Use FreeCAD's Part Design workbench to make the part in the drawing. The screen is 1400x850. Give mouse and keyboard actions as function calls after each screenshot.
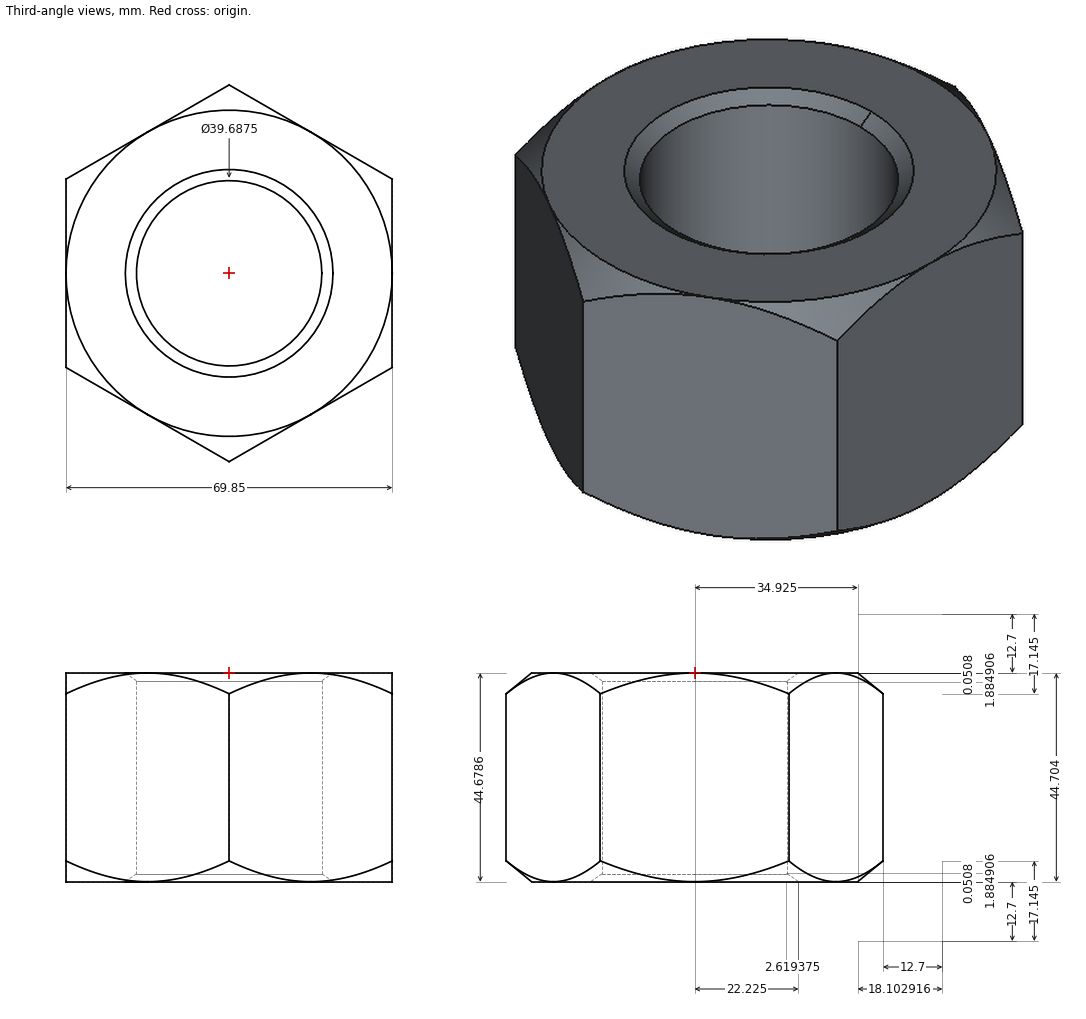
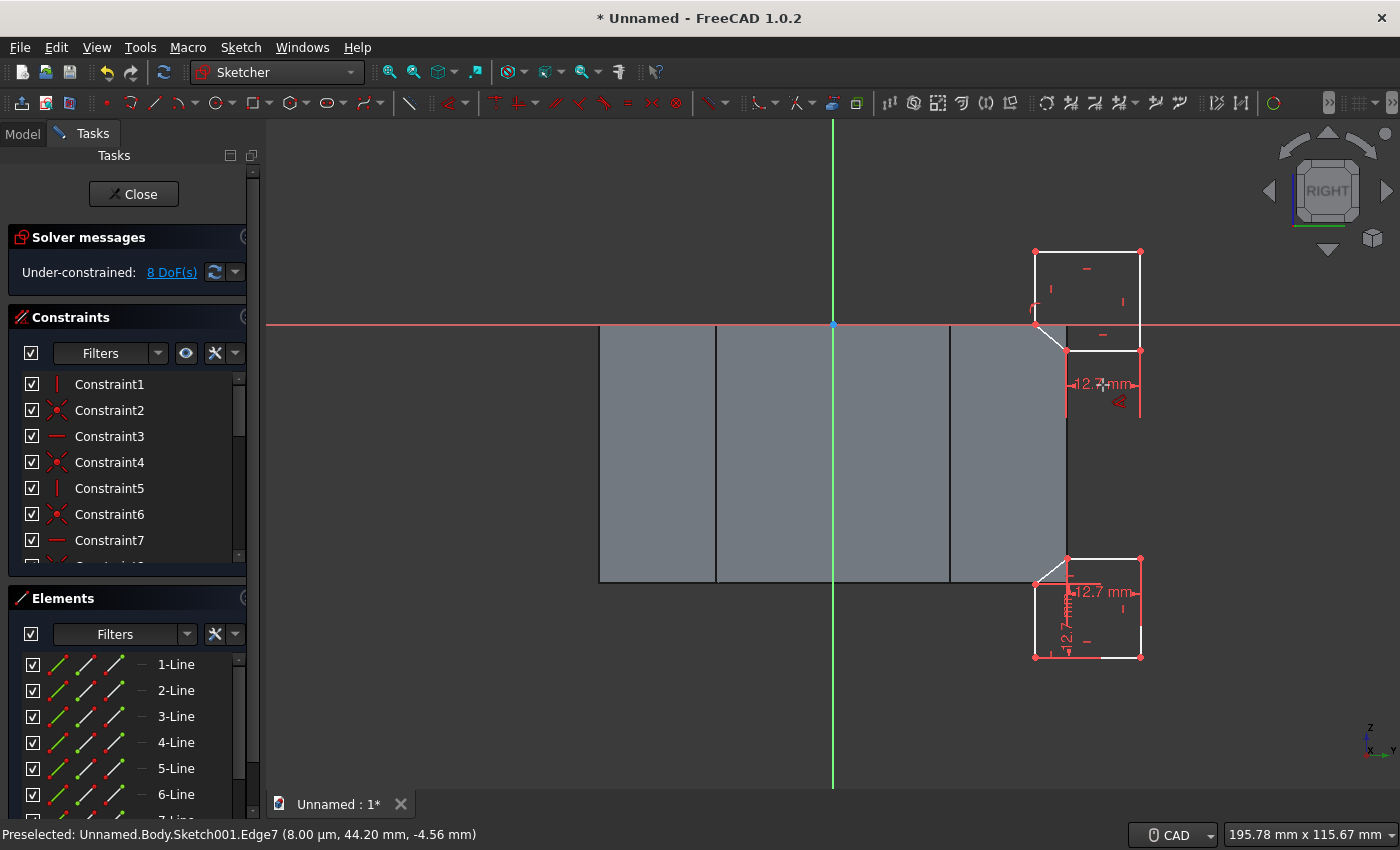
click(1035, 274)
click(1069, 288)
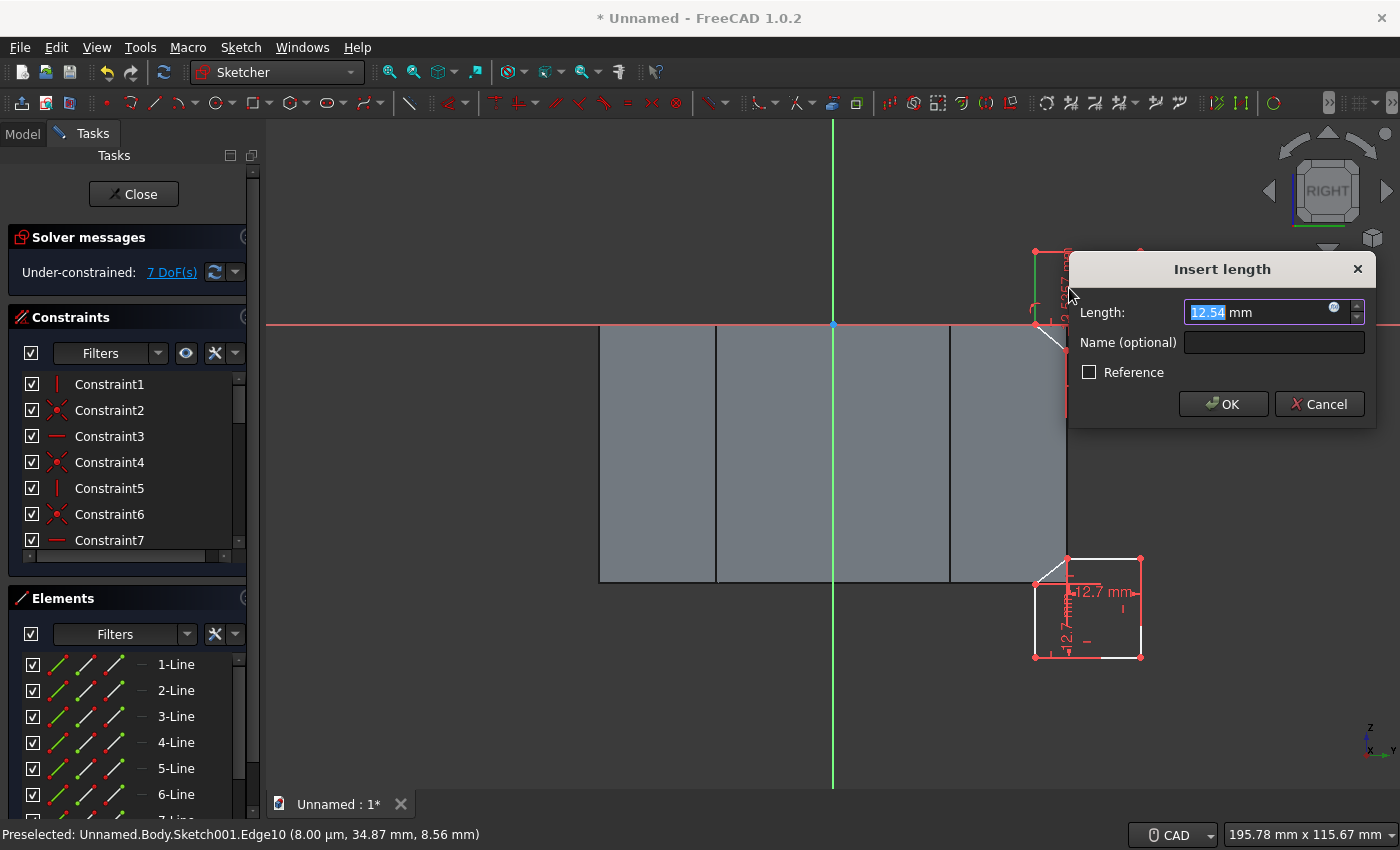
text(12.7)
key(Return)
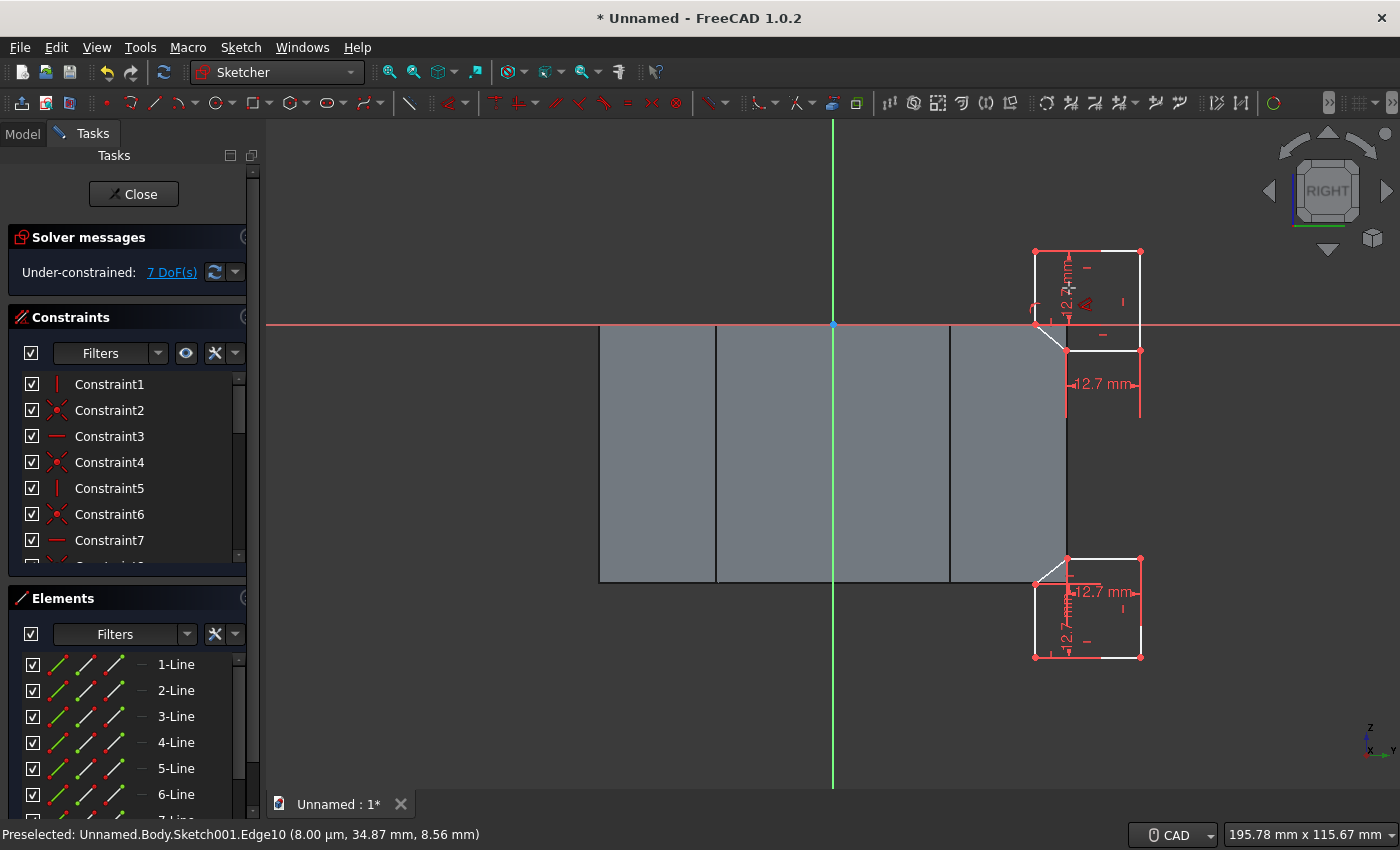
click(1141, 628)
click(1175, 608)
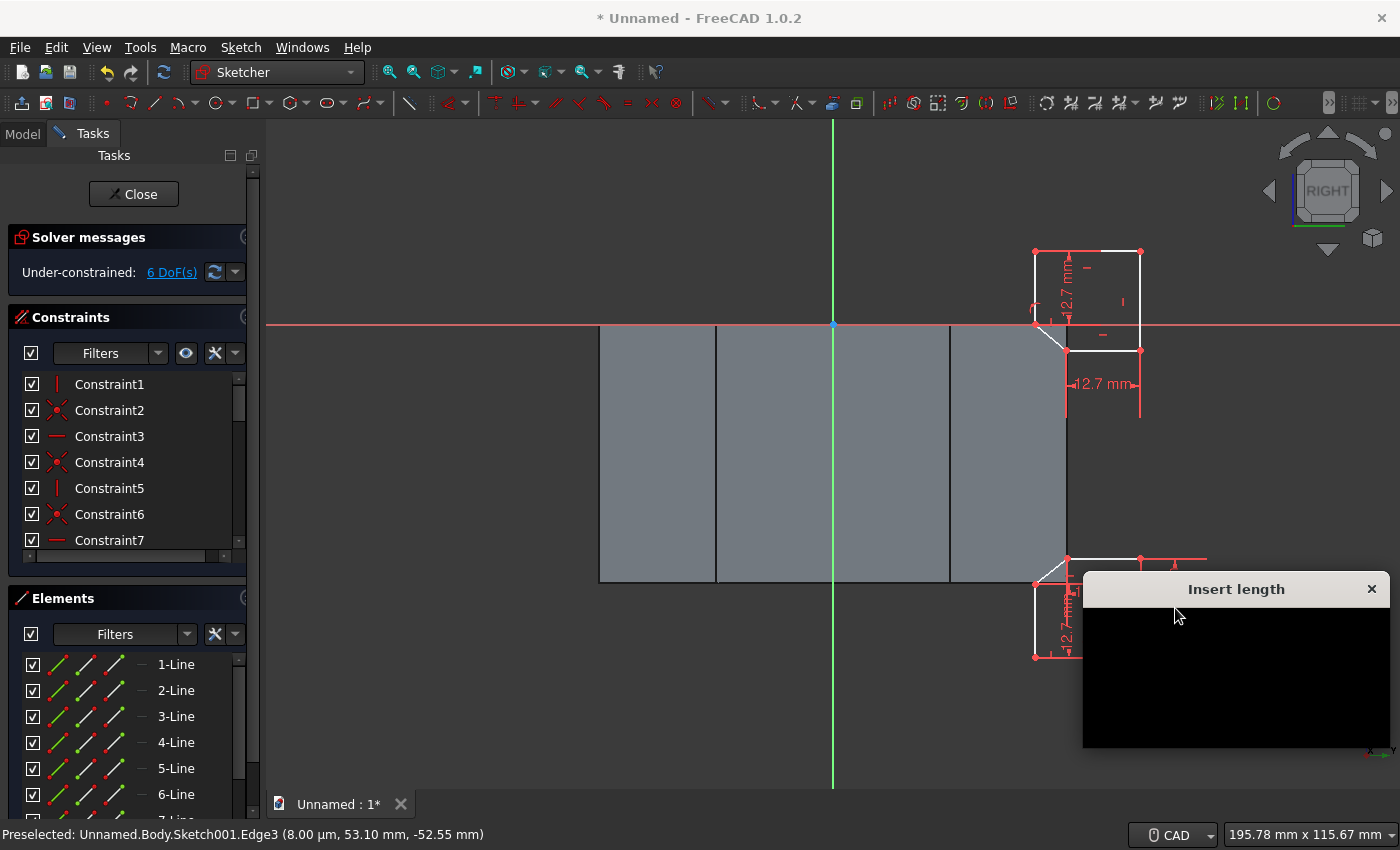
text(17.145)
key(Return)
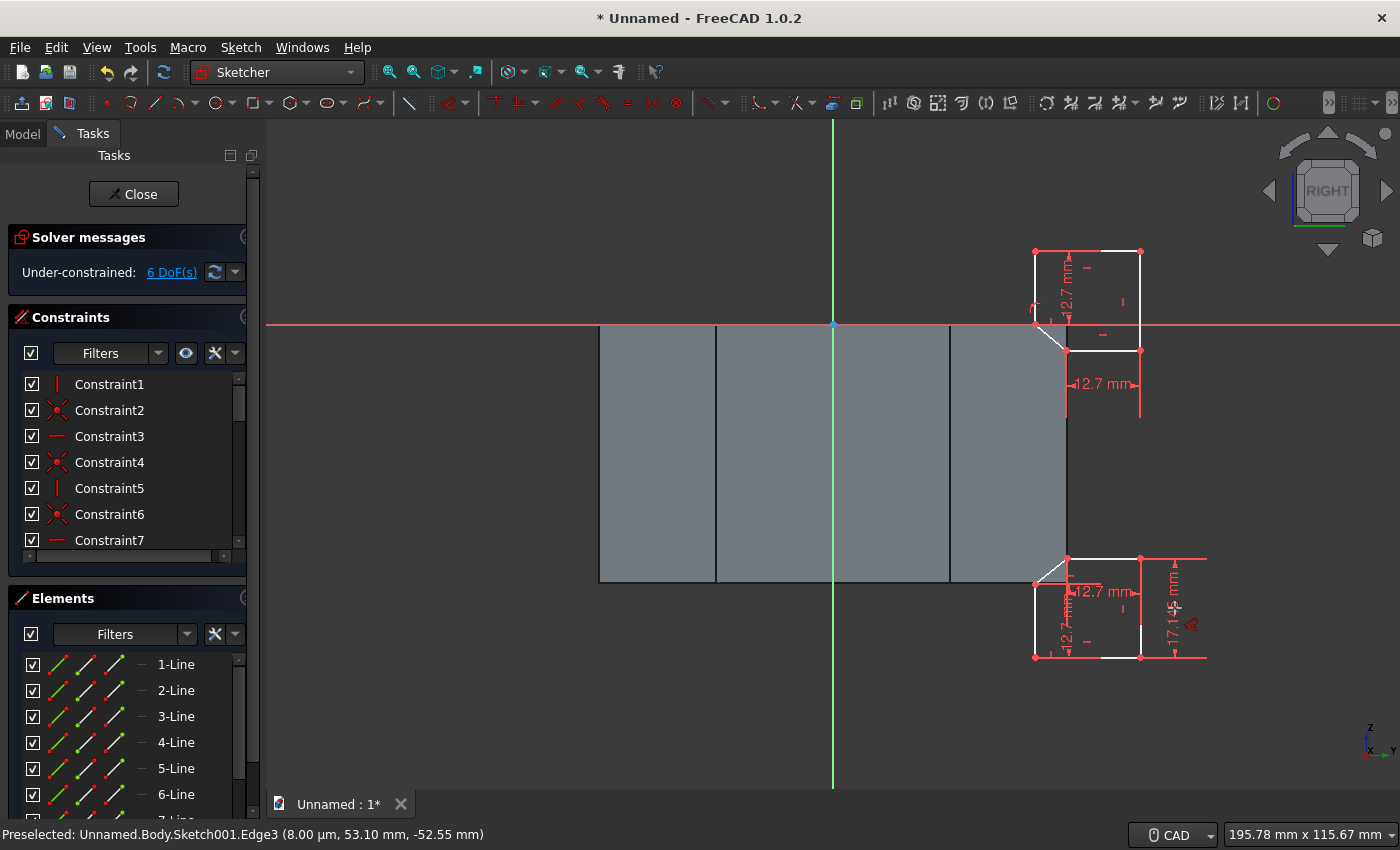
click(1140, 321)
click(1174, 301)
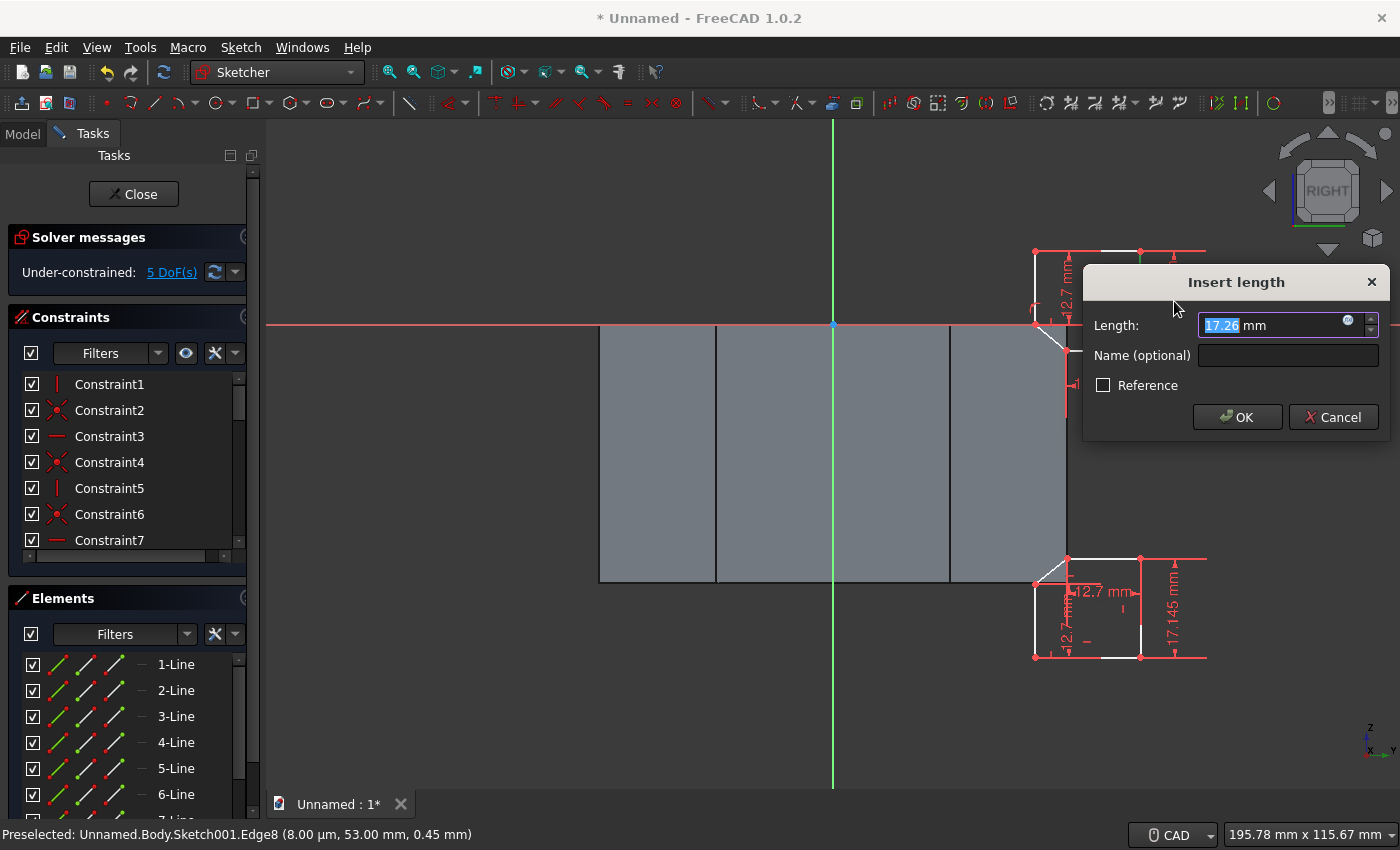
text(17.145)
key(Return)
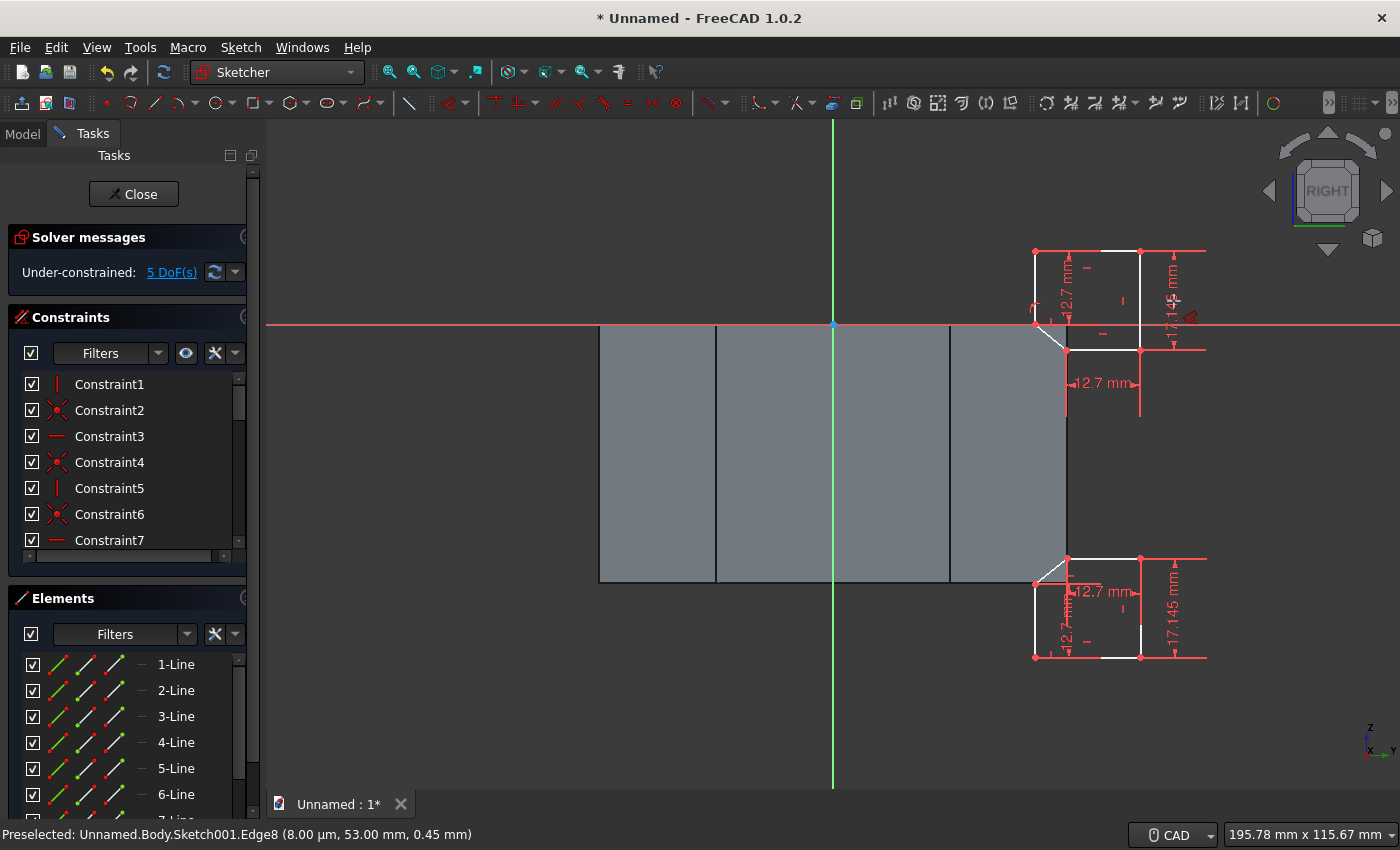
click(1035, 584)
click(934, 618)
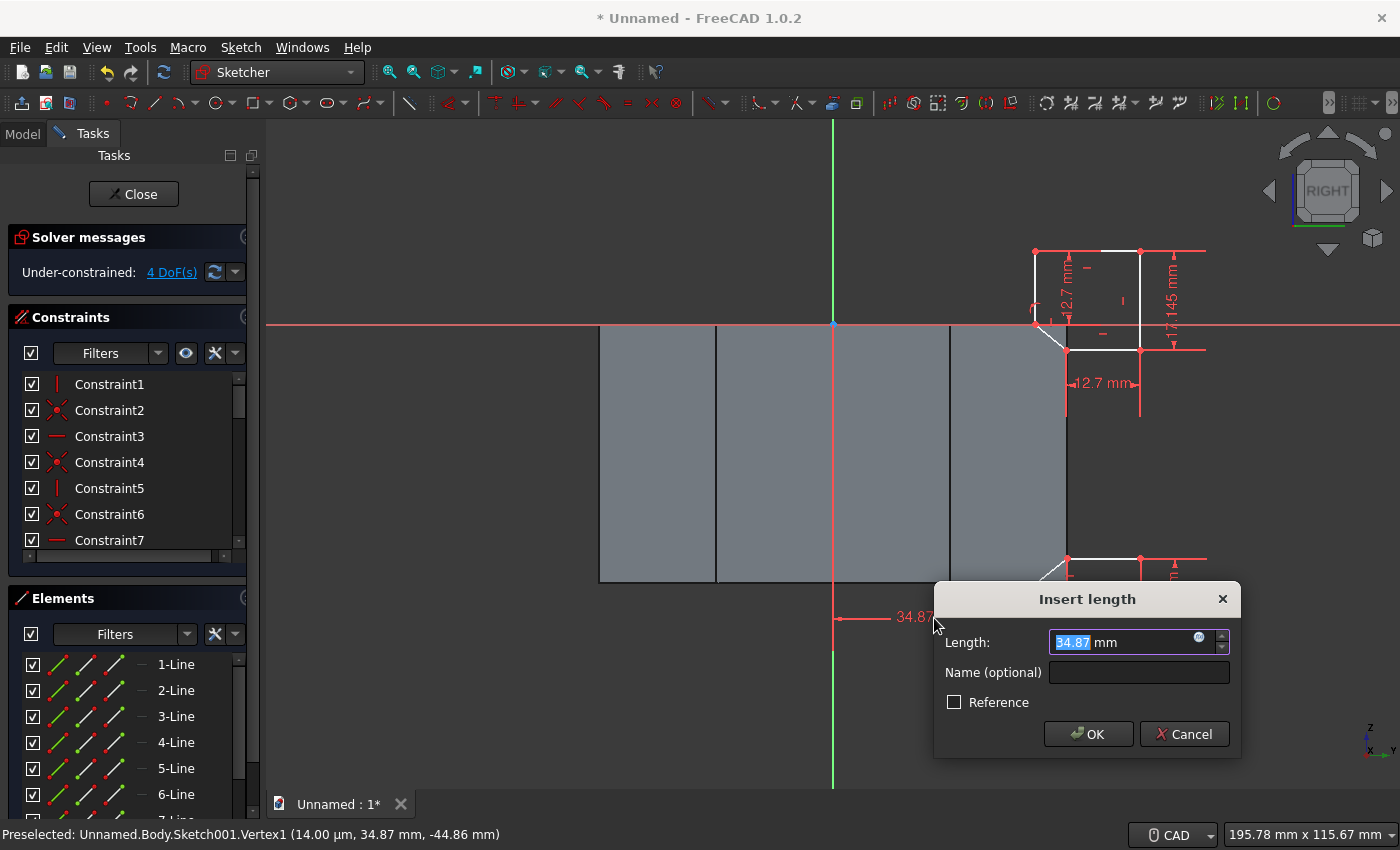
text(34.925)
key(Return)